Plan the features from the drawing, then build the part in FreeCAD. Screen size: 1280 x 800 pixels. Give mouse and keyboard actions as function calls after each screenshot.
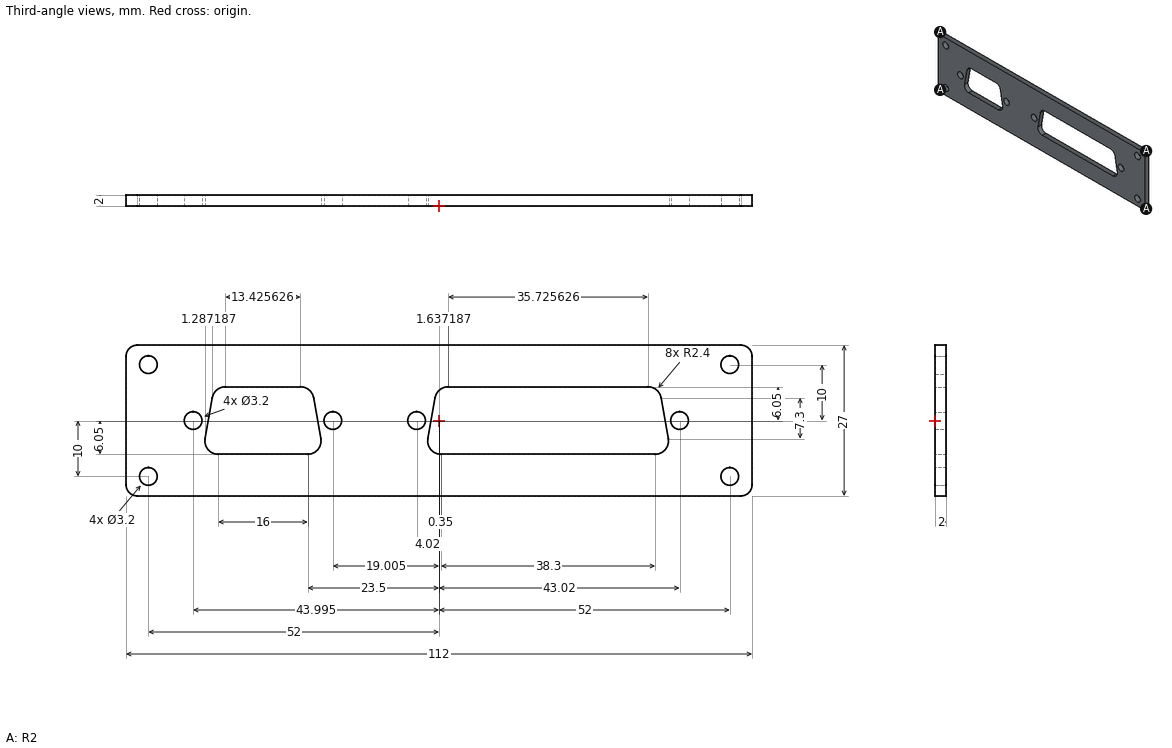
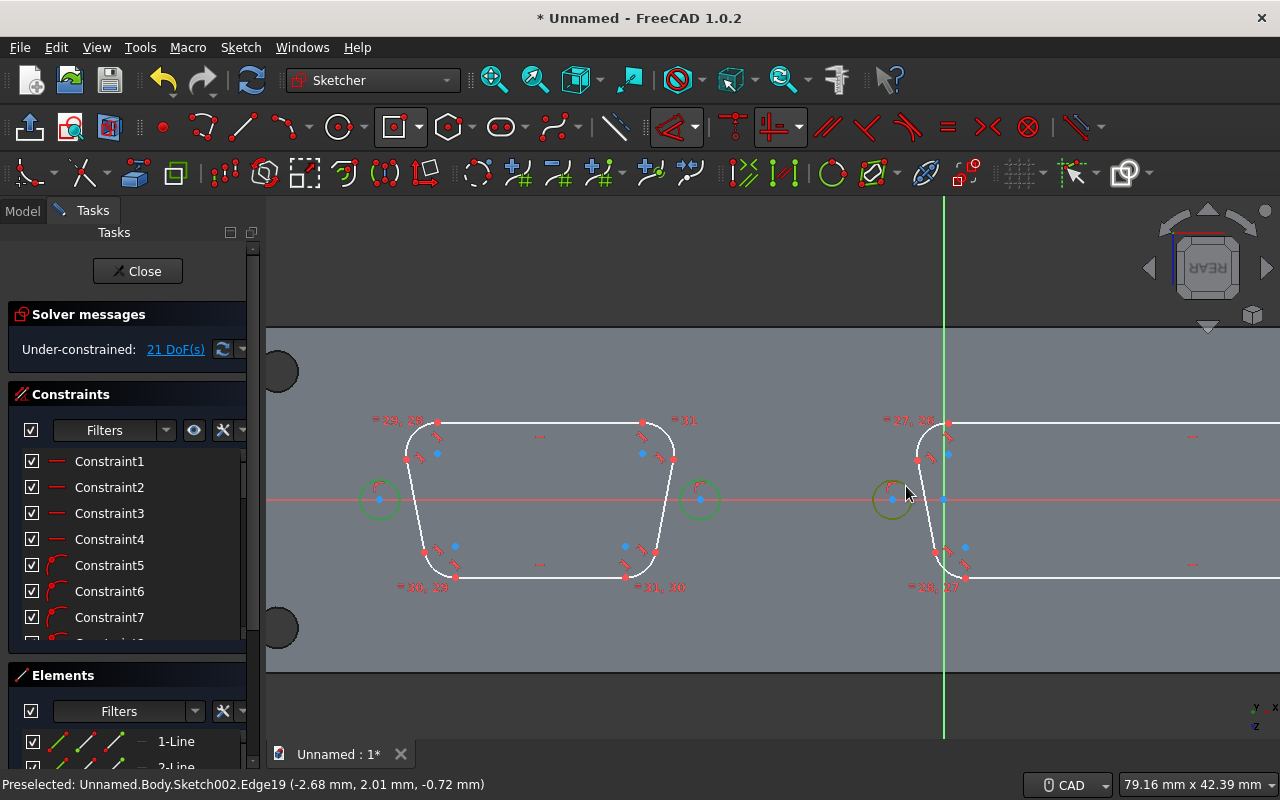
scroll(421, 428, down, 3)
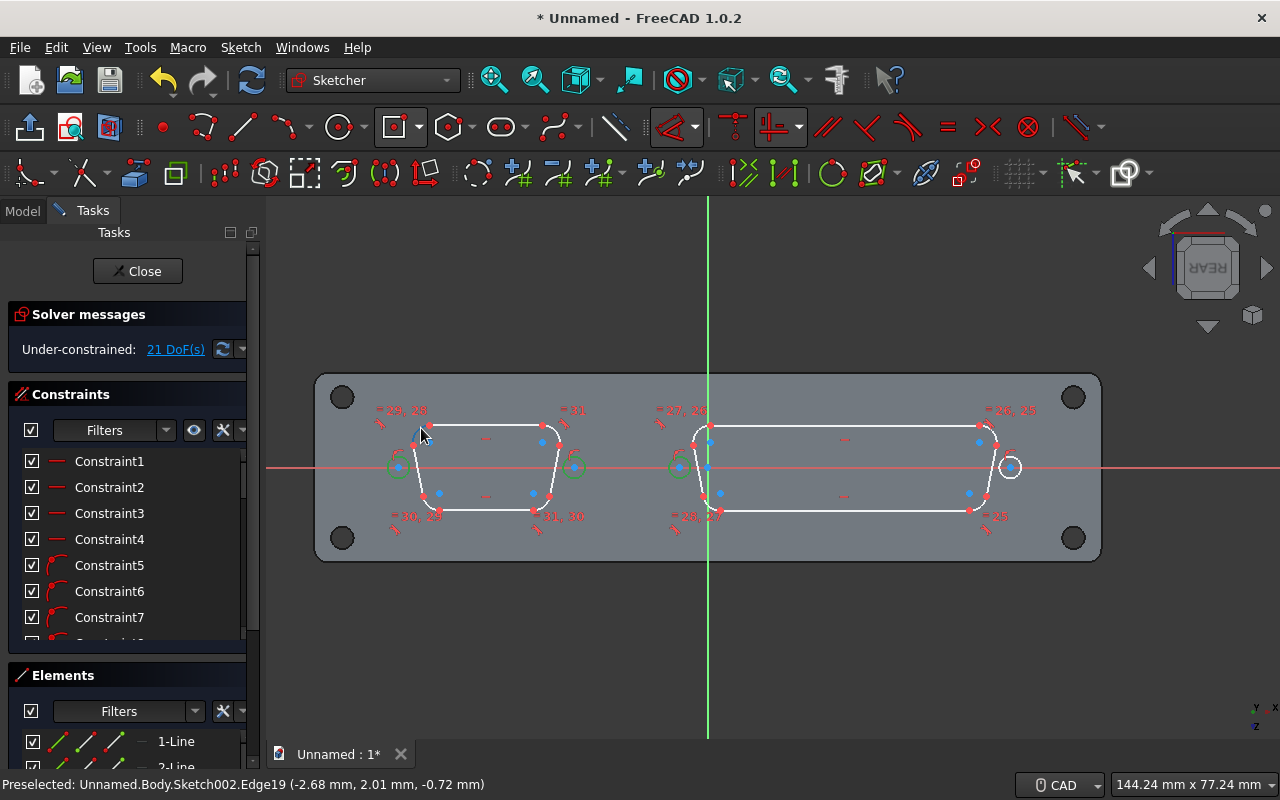
scroll(1018, 460, up, 3)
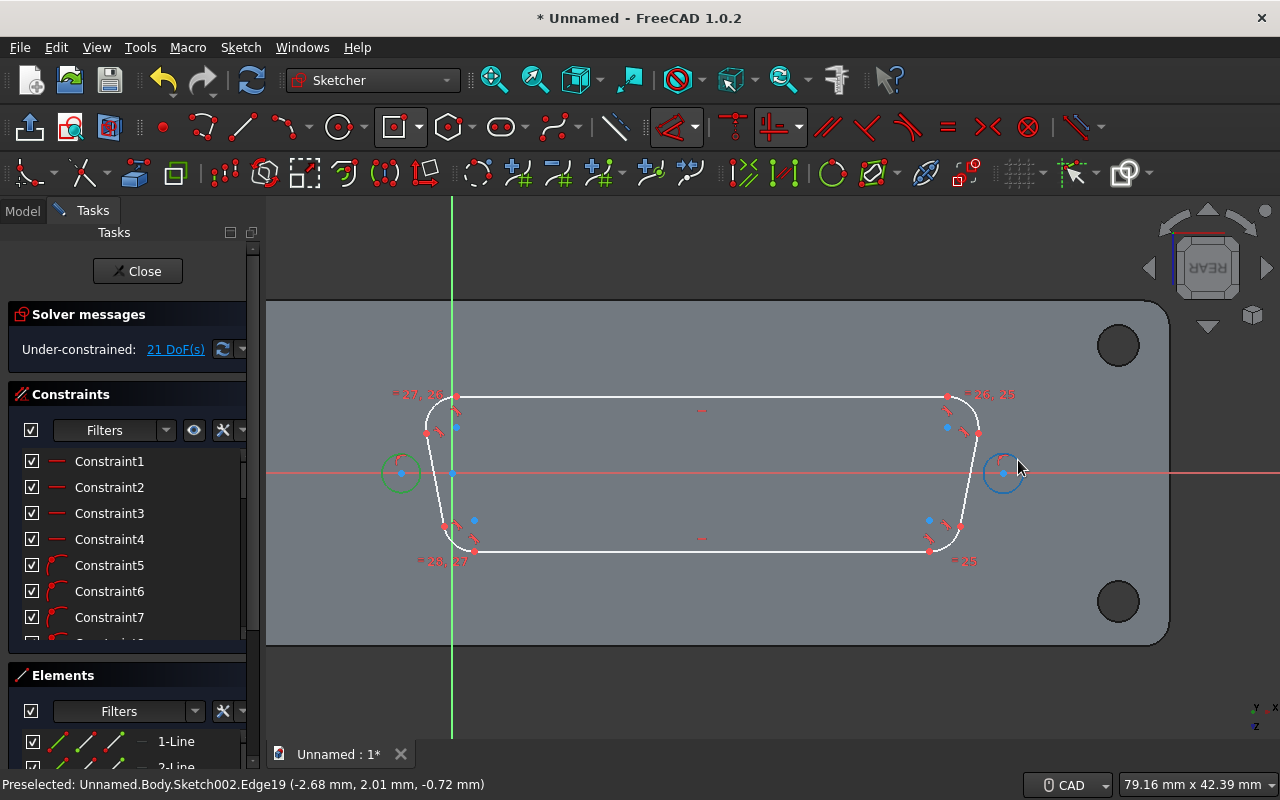
click(1017, 459)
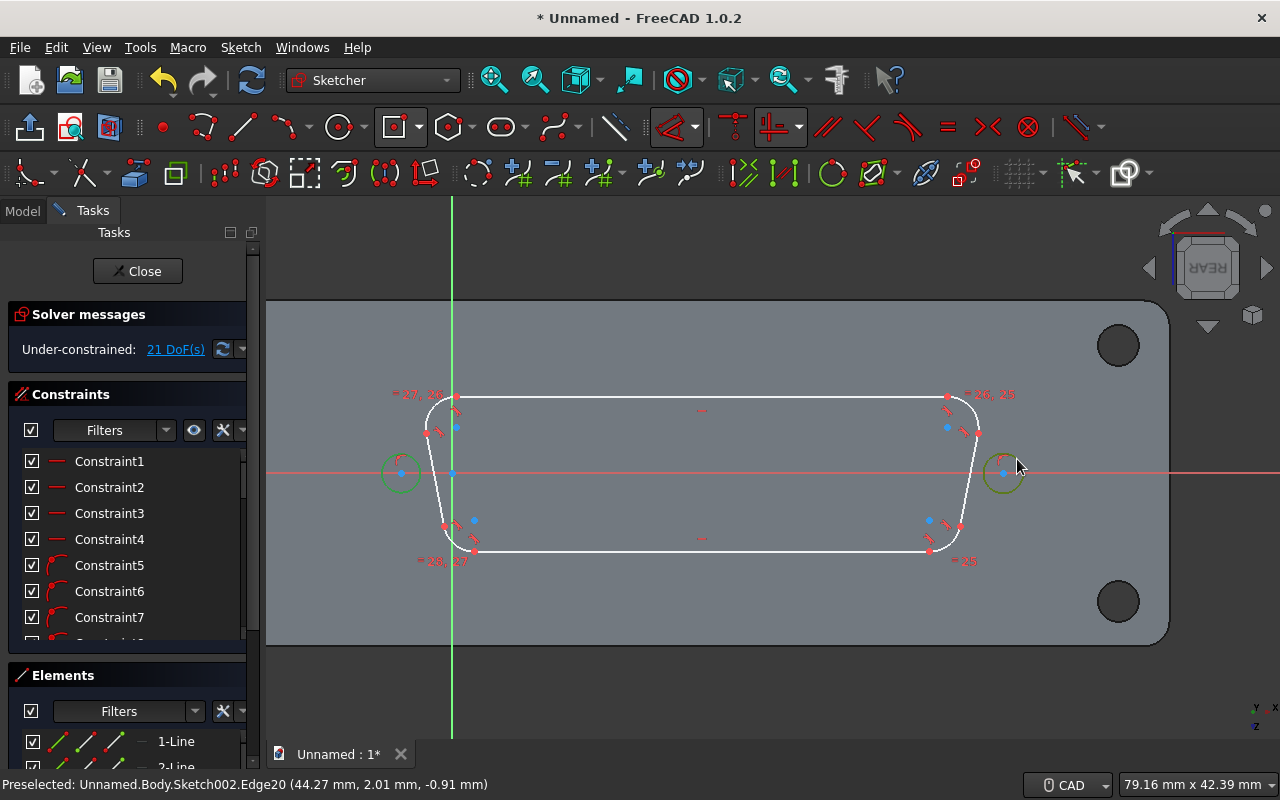
click(948, 128)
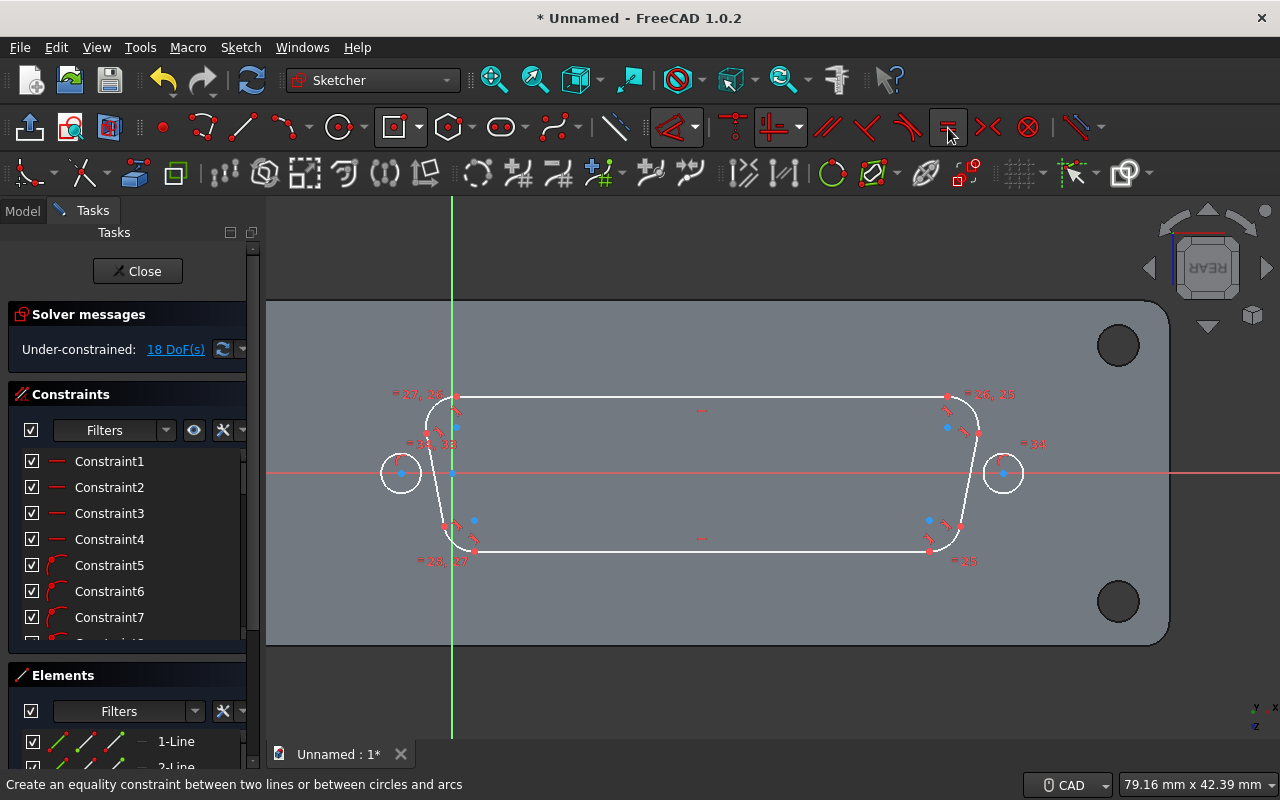
scroll(942, 549, up, 2)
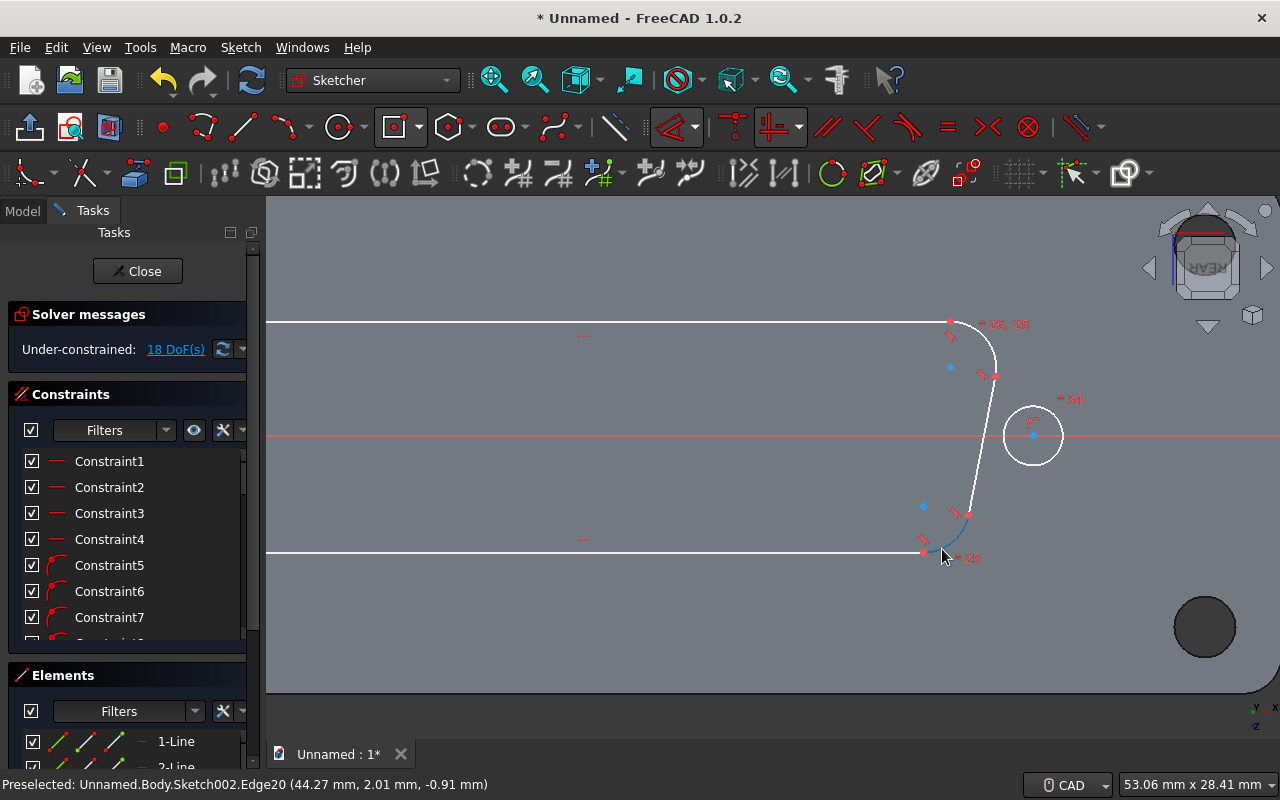
click(942, 549)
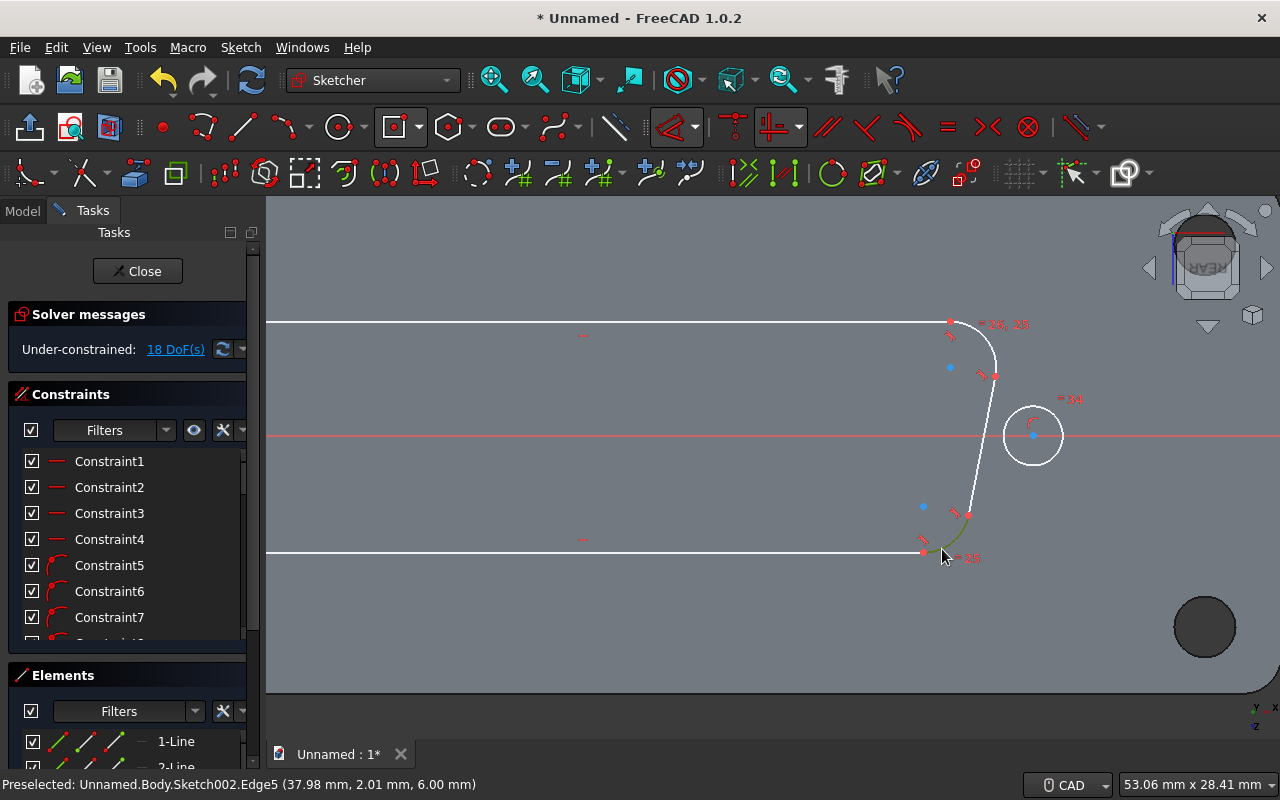
click(698, 128)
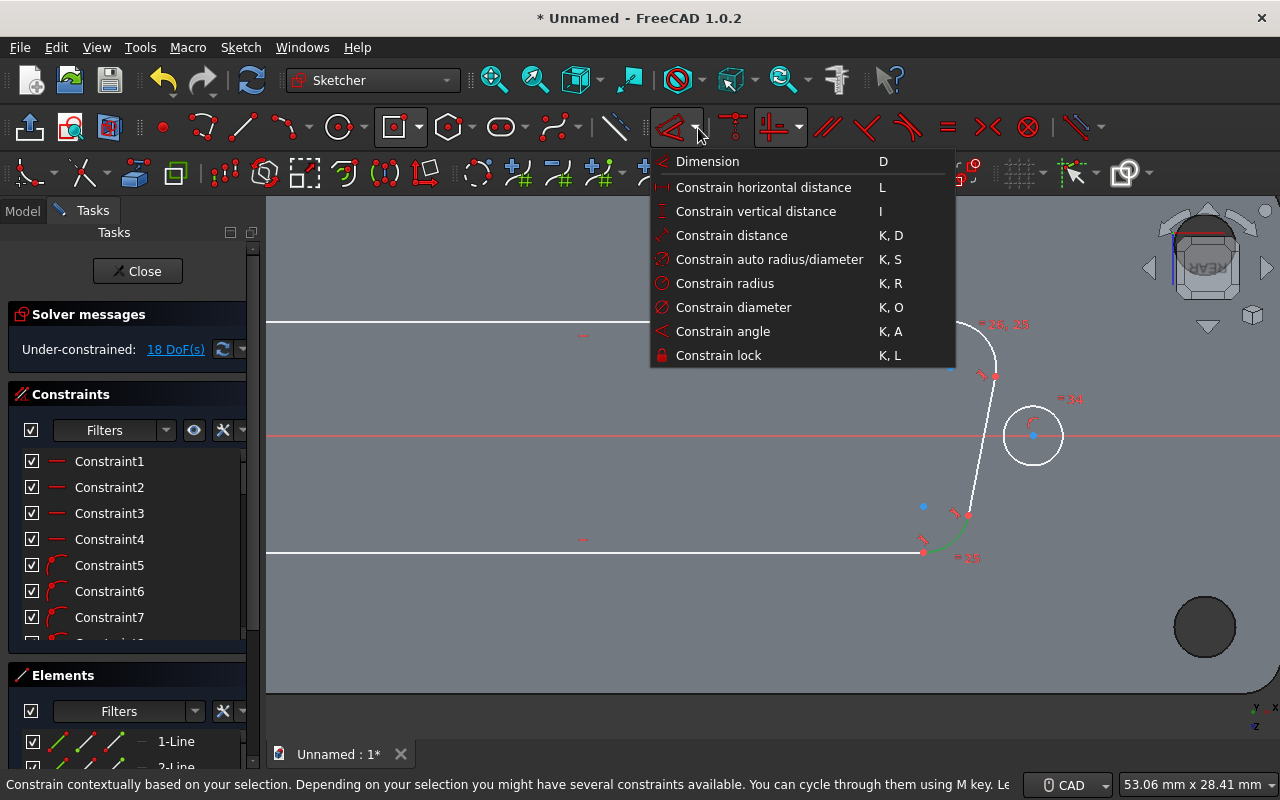
click(803, 283)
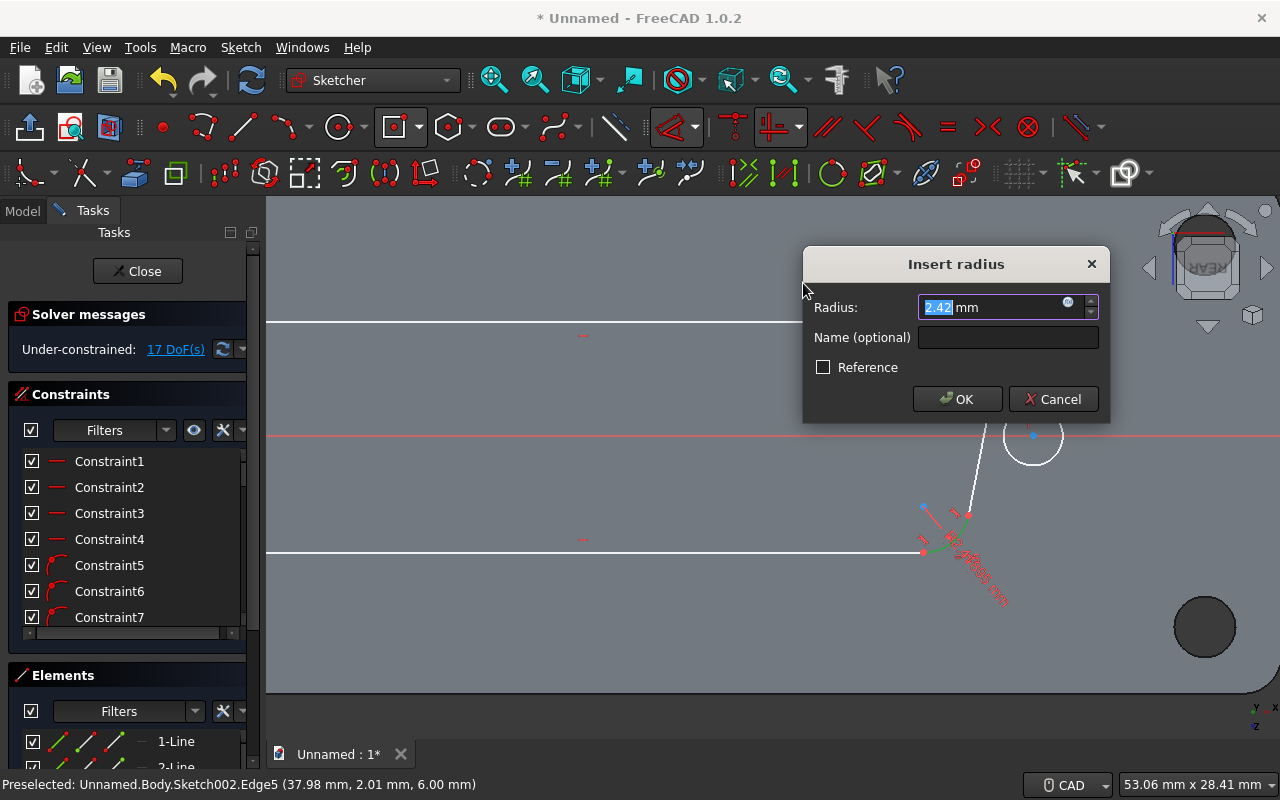
text(2.4)
key(Return)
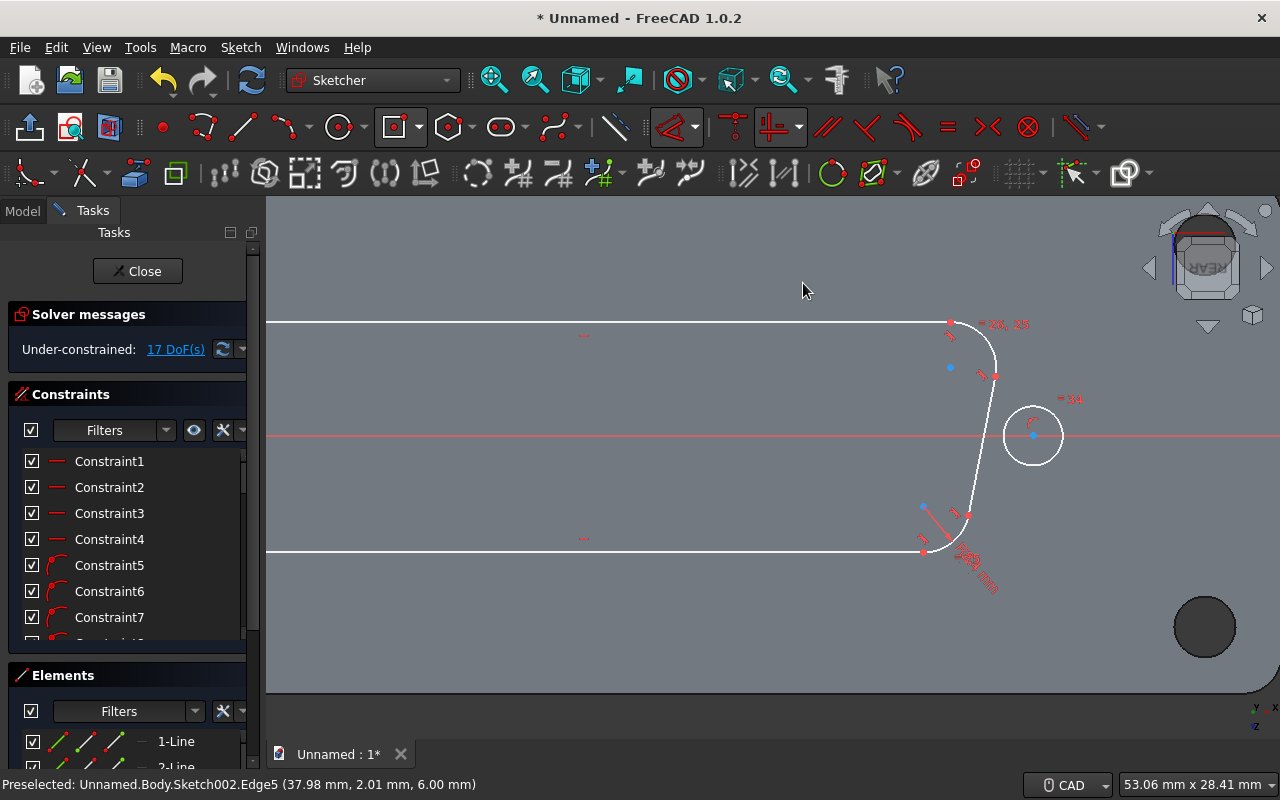
scroll(997, 486, down, 5)